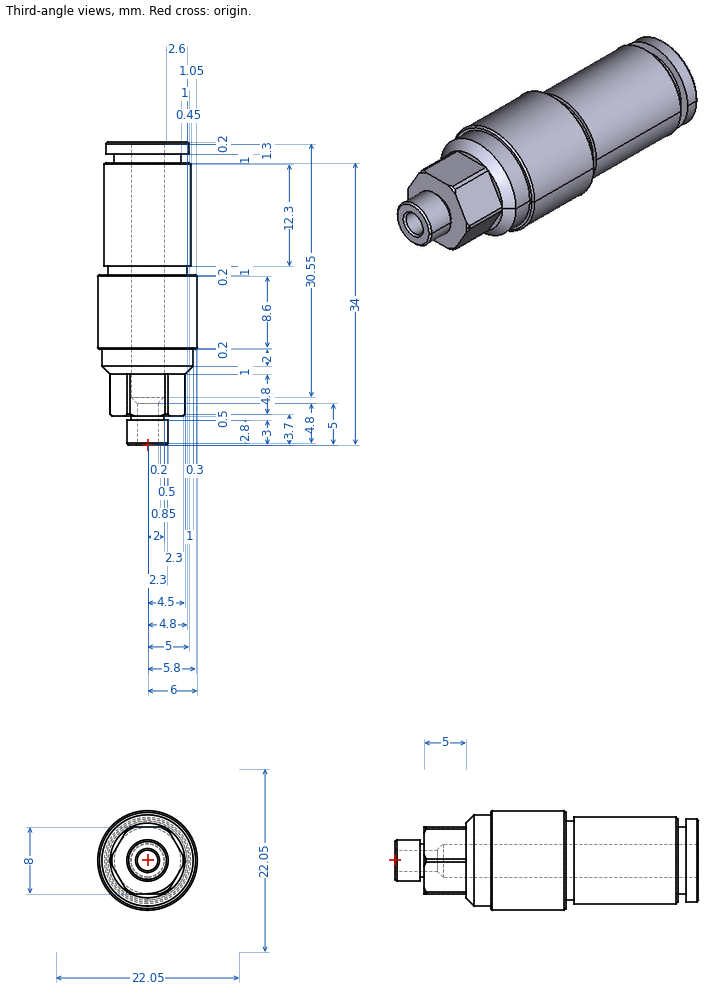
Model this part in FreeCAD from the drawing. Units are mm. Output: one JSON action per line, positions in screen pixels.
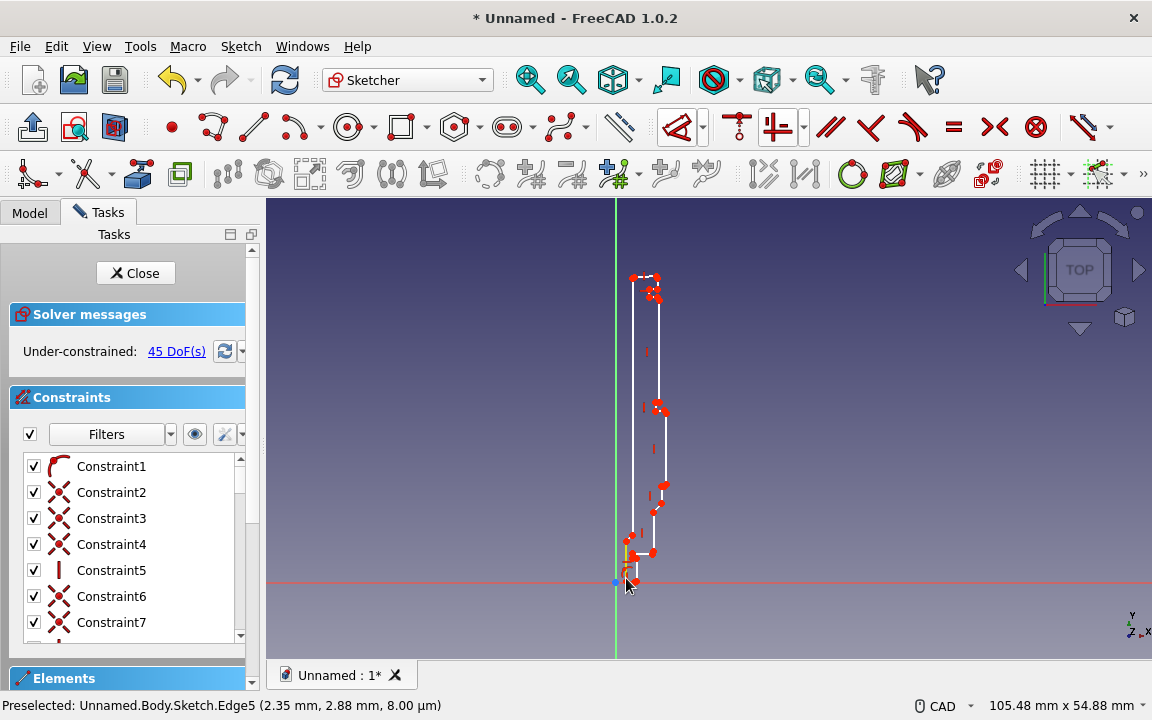
{"action": "scroll", "coordinate": [639, 554], "scroll_direction": "up", "scroll_amount": 5}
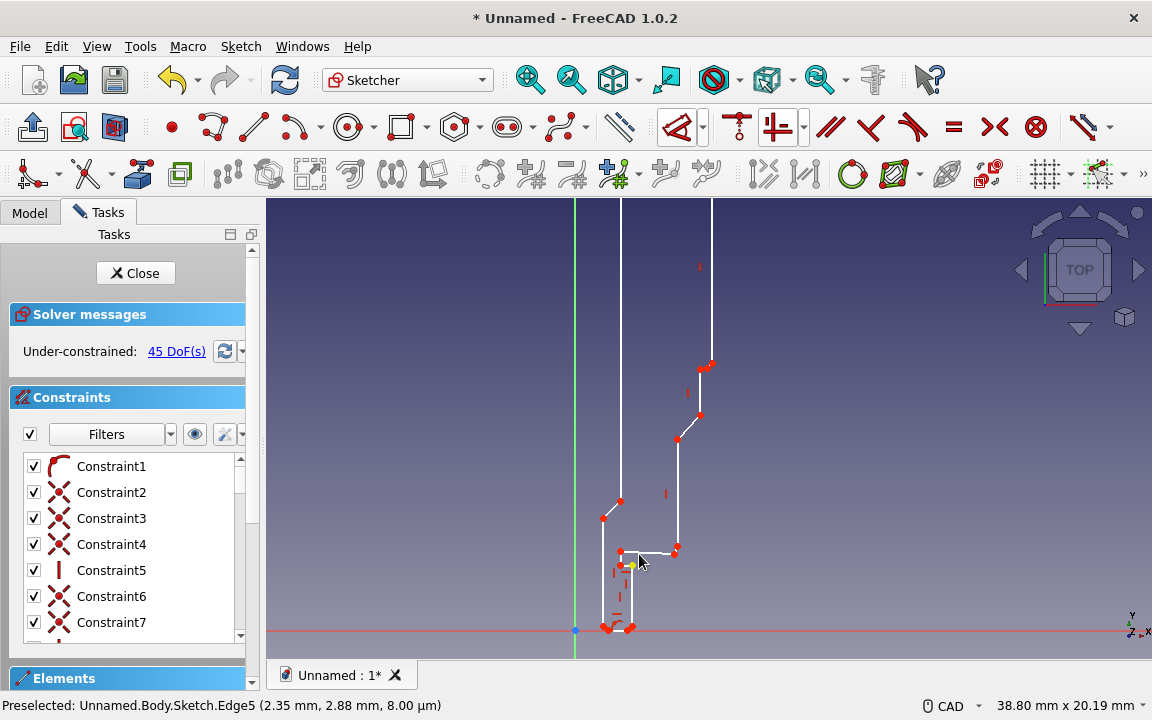
{"action": "left_click", "coordinate": [637, 552]}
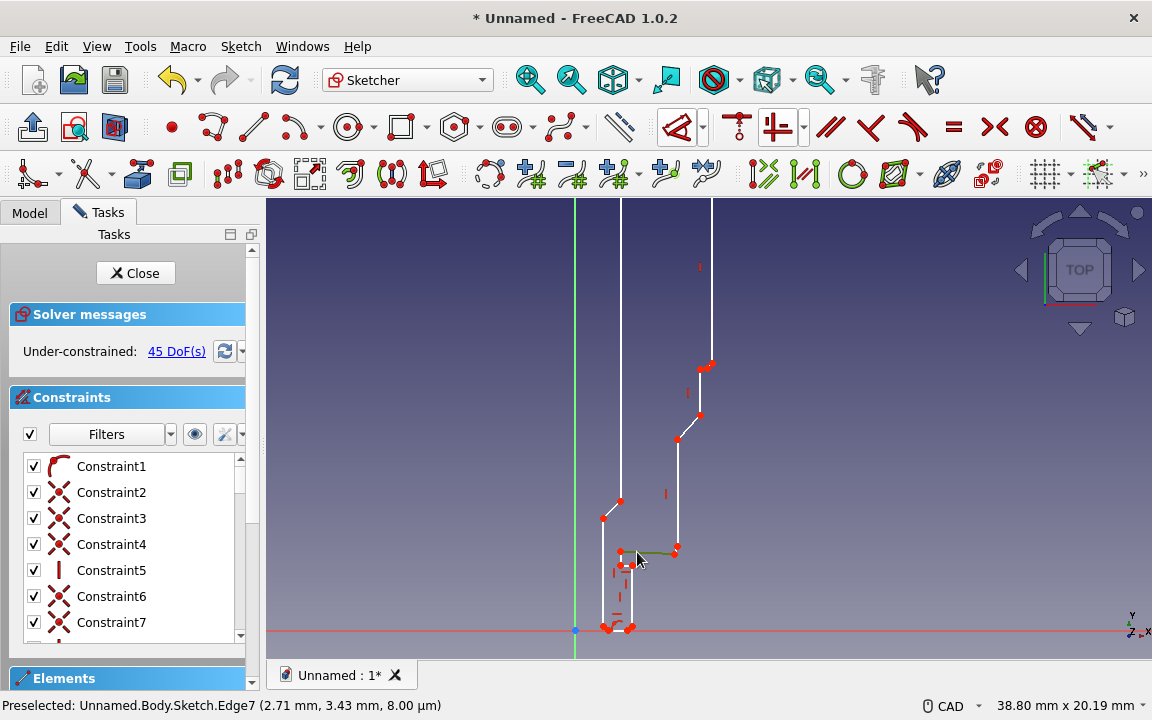
{"action": "left_click", "coordinate": [804, 128]}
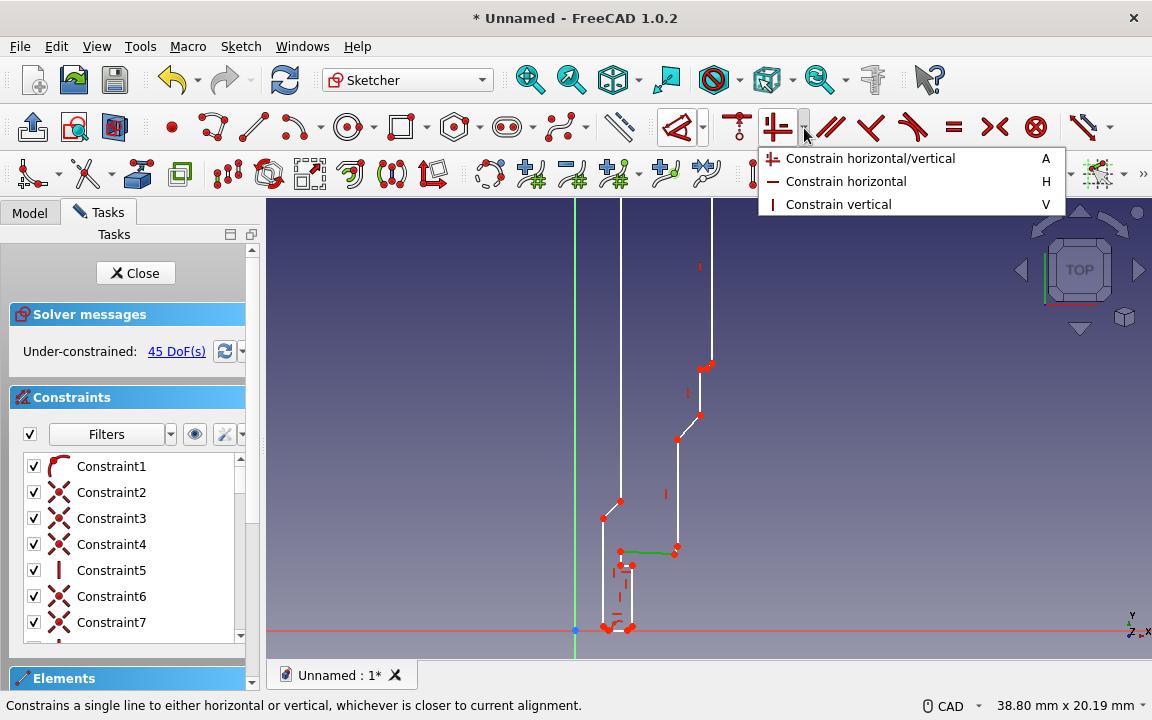
{"action": "left_click", "coordinate": [912, 182]}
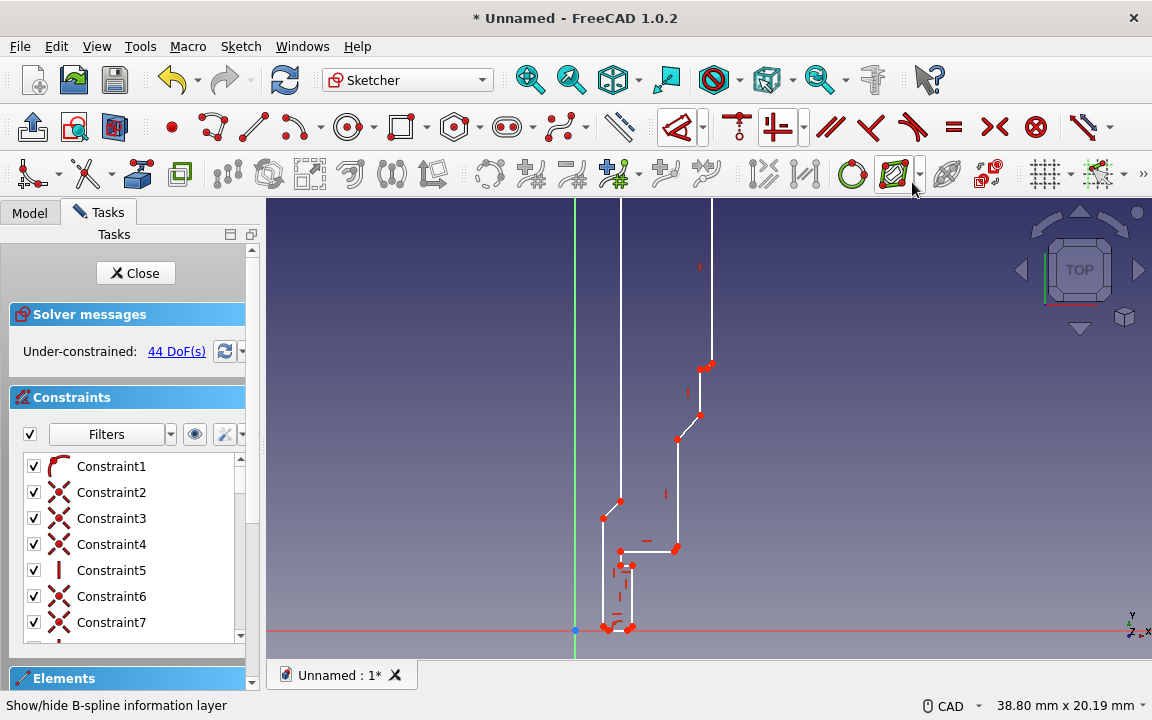
{"action": "scroll", "coordinate": [704, 369], "scroll_direction": "up", "scroll_amount": 7}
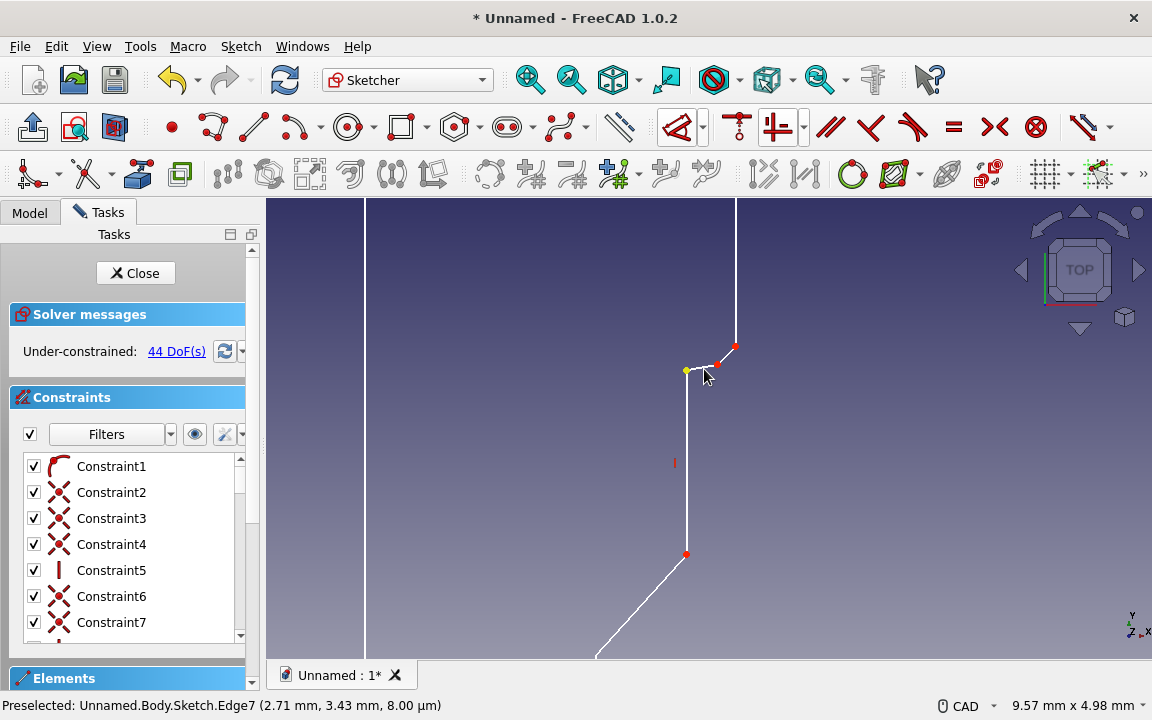
{"action": "left_click", "coordinate": [702, 367]}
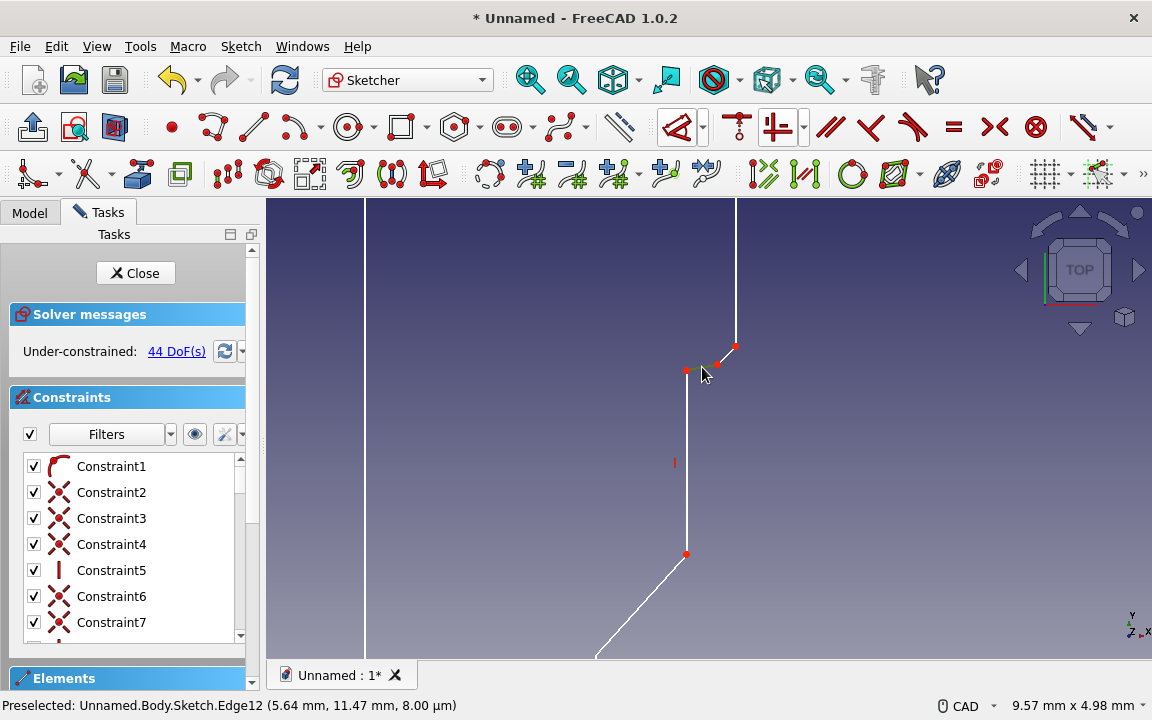
{"action": "left_click", "coordinate": [804, 128]}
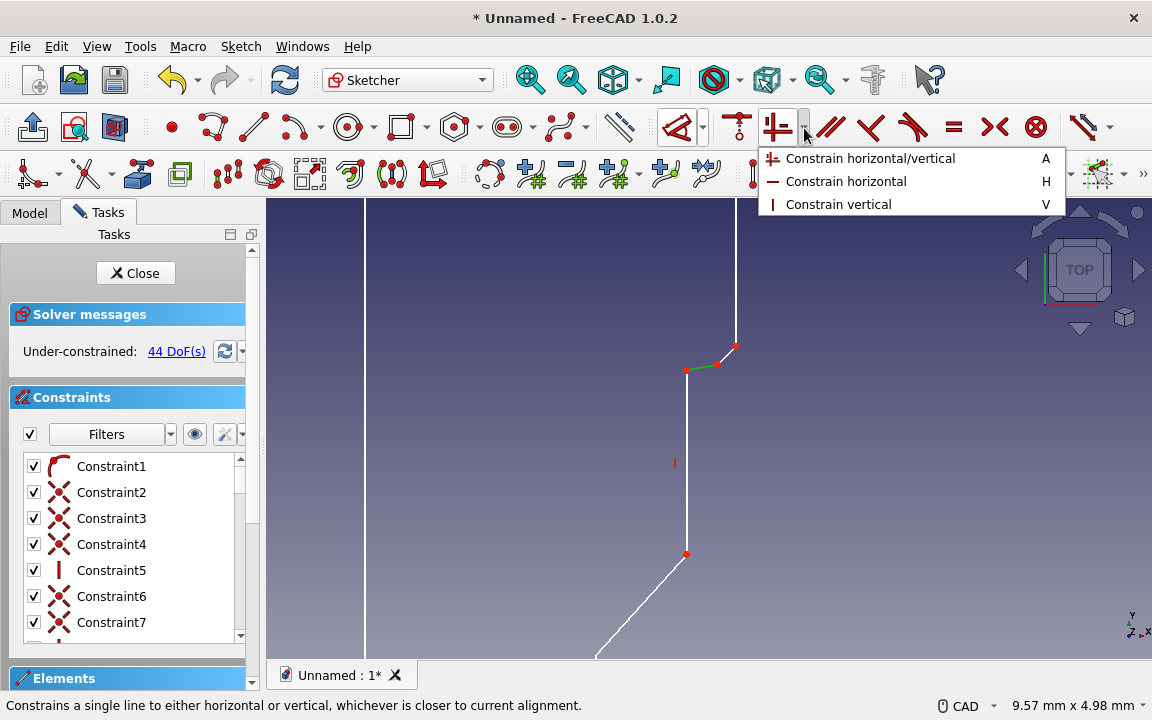
{"action": "left_click", "coordinate": [912, 182]}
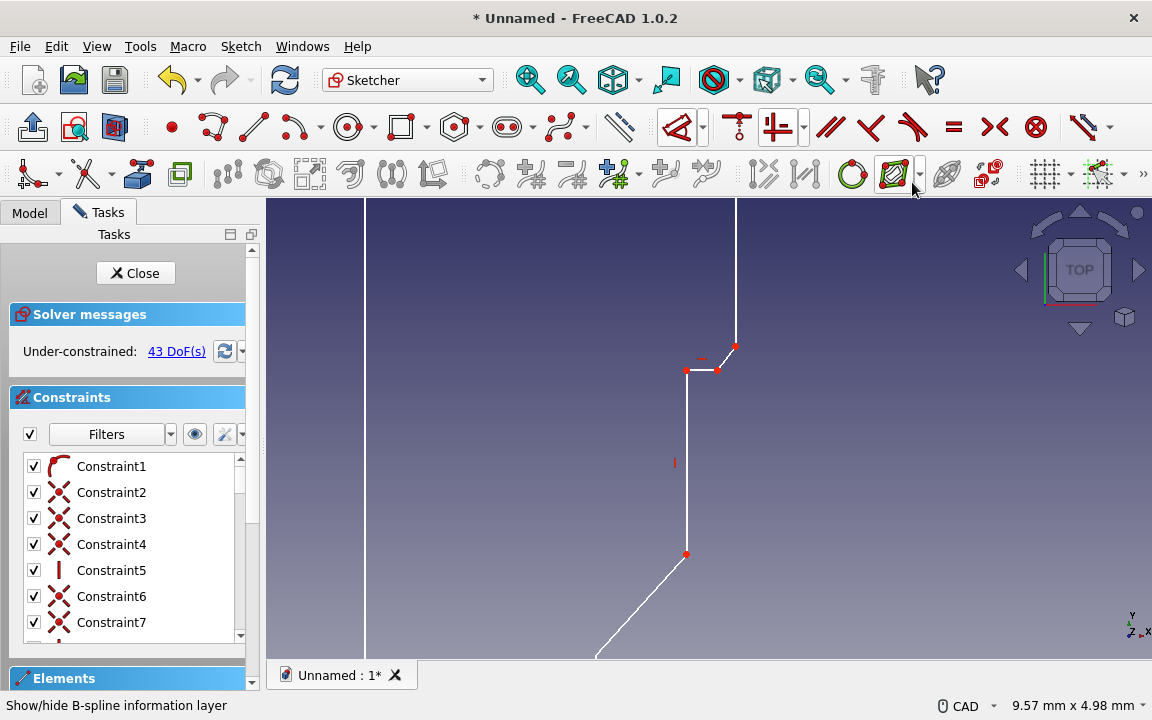
{"action": "scroll", "coordinate": [659, 497], "scroll_direction": "down", "scroll_amount": 12}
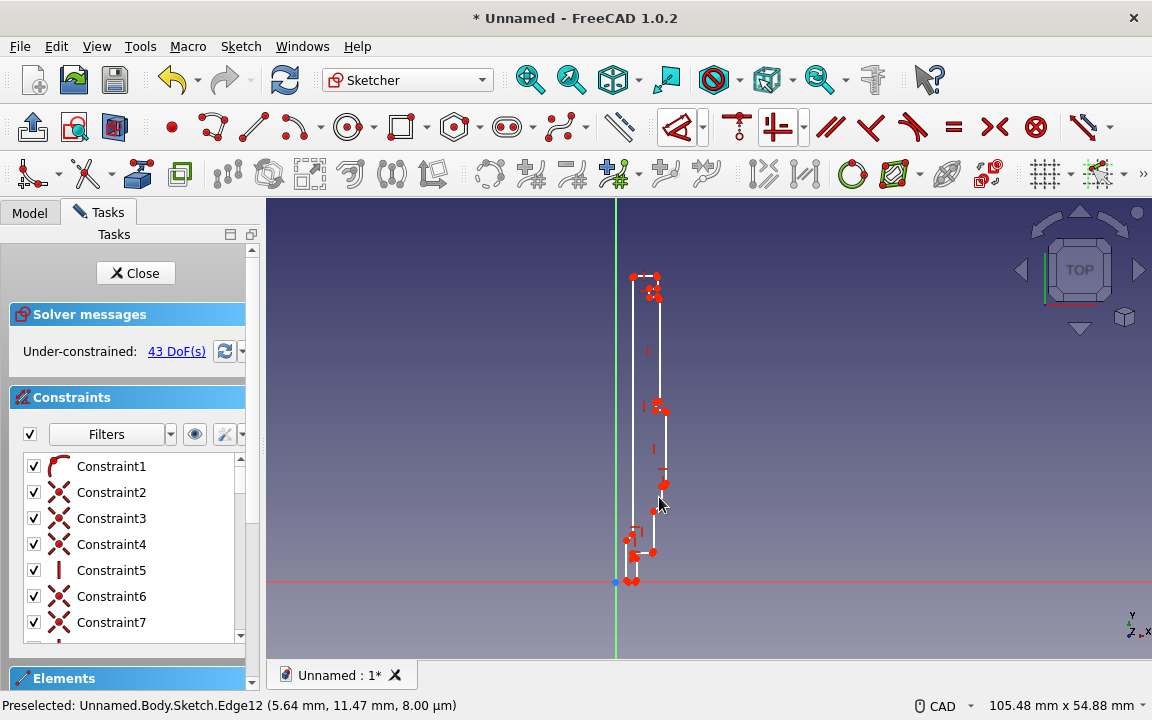
{"action": "scroll", "coordinate": [662, 410], "scroll_direction": "up", "scroll_amount": 9}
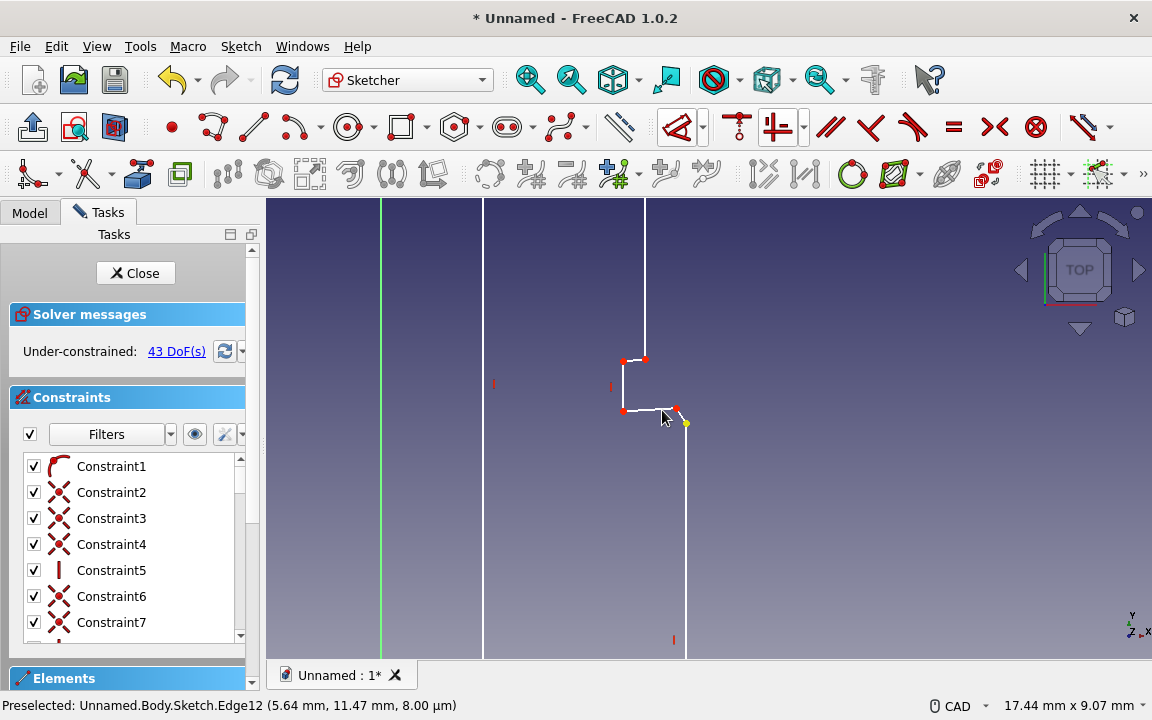
{"action": "left_click", "coordinate": [660, 409]}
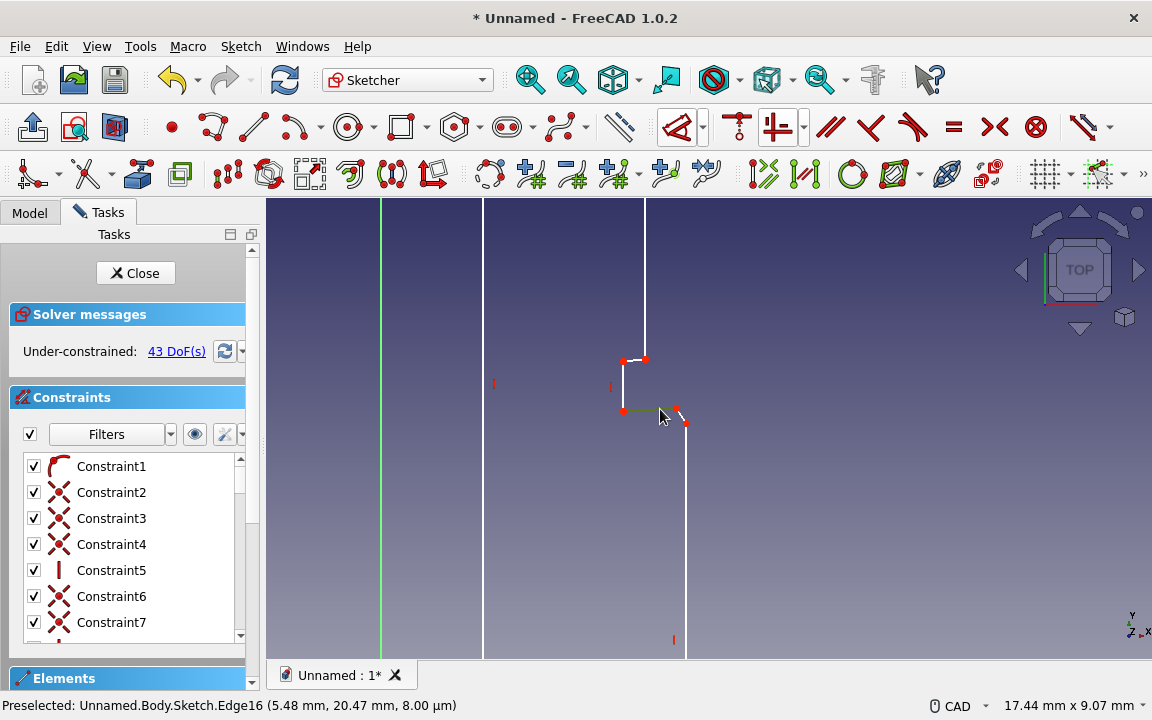
{"action": "left_click", "coordinate": [804, 128]}